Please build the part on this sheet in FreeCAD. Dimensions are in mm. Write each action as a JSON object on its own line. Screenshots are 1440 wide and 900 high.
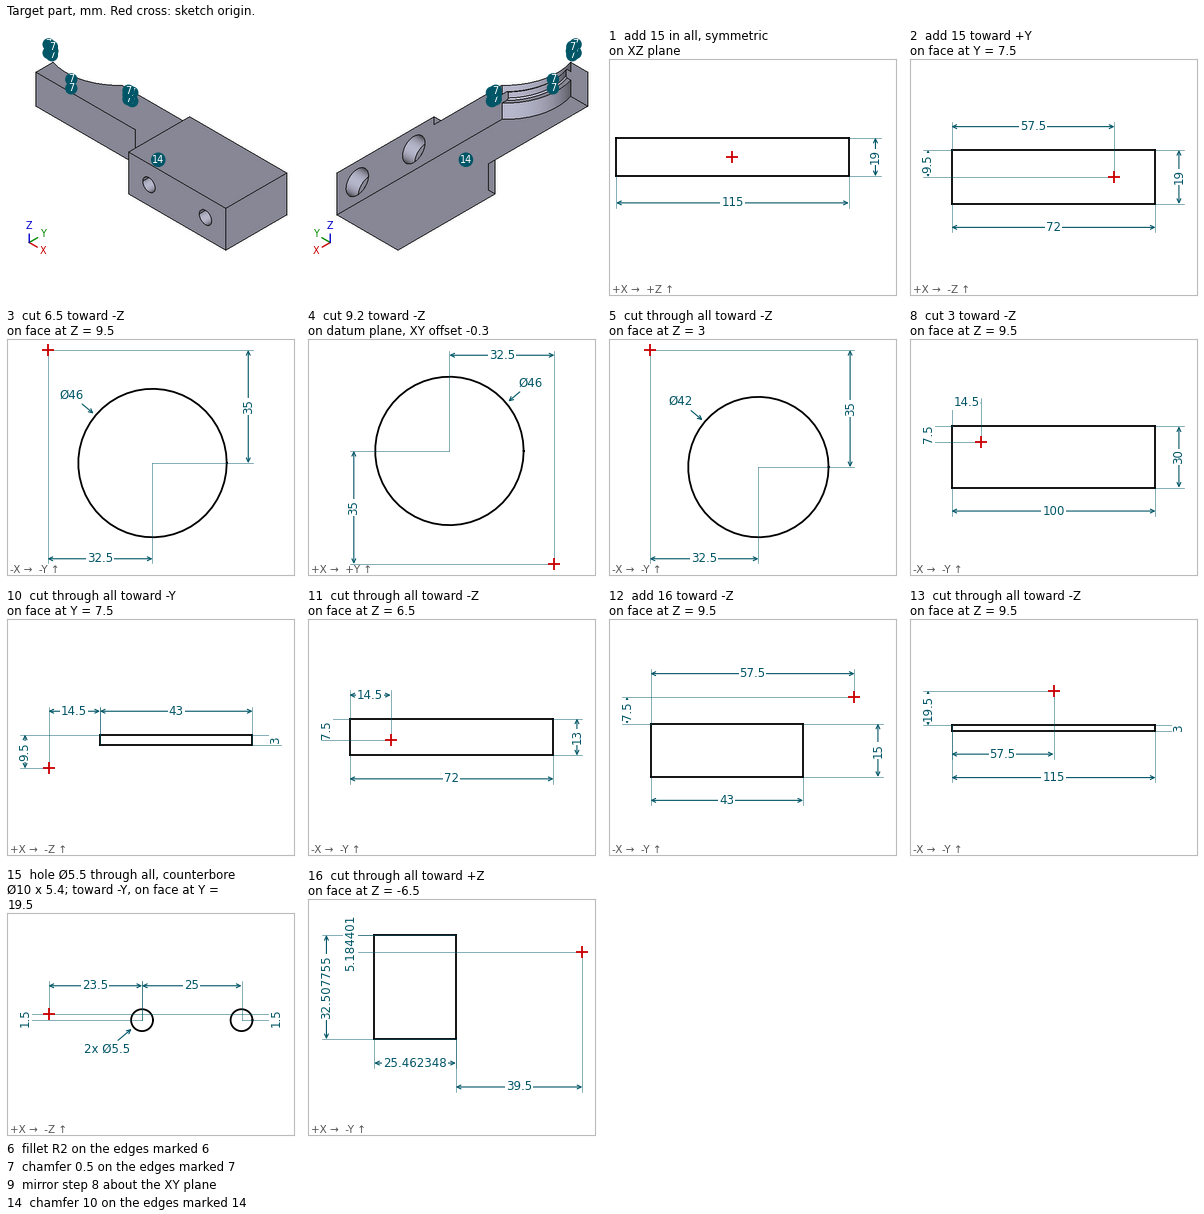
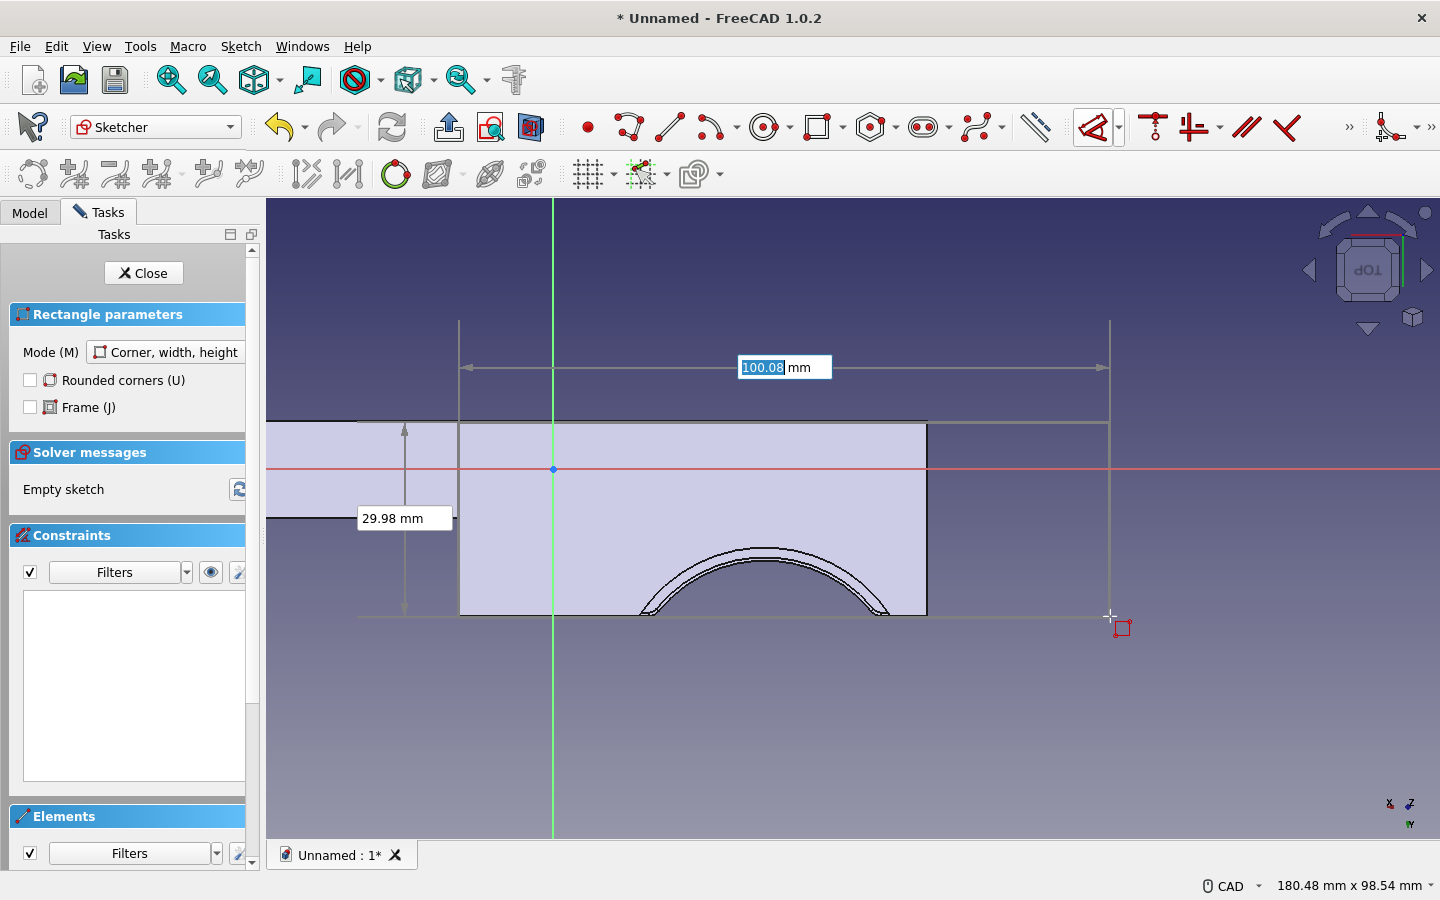
{"action": "type", "text": "100"}
{"action": "key", "text": "Tab"}
{"action": "type", "text": "30"}
{"action": "key", "text": "Return"}
{"action": "key", "text": "Escape"}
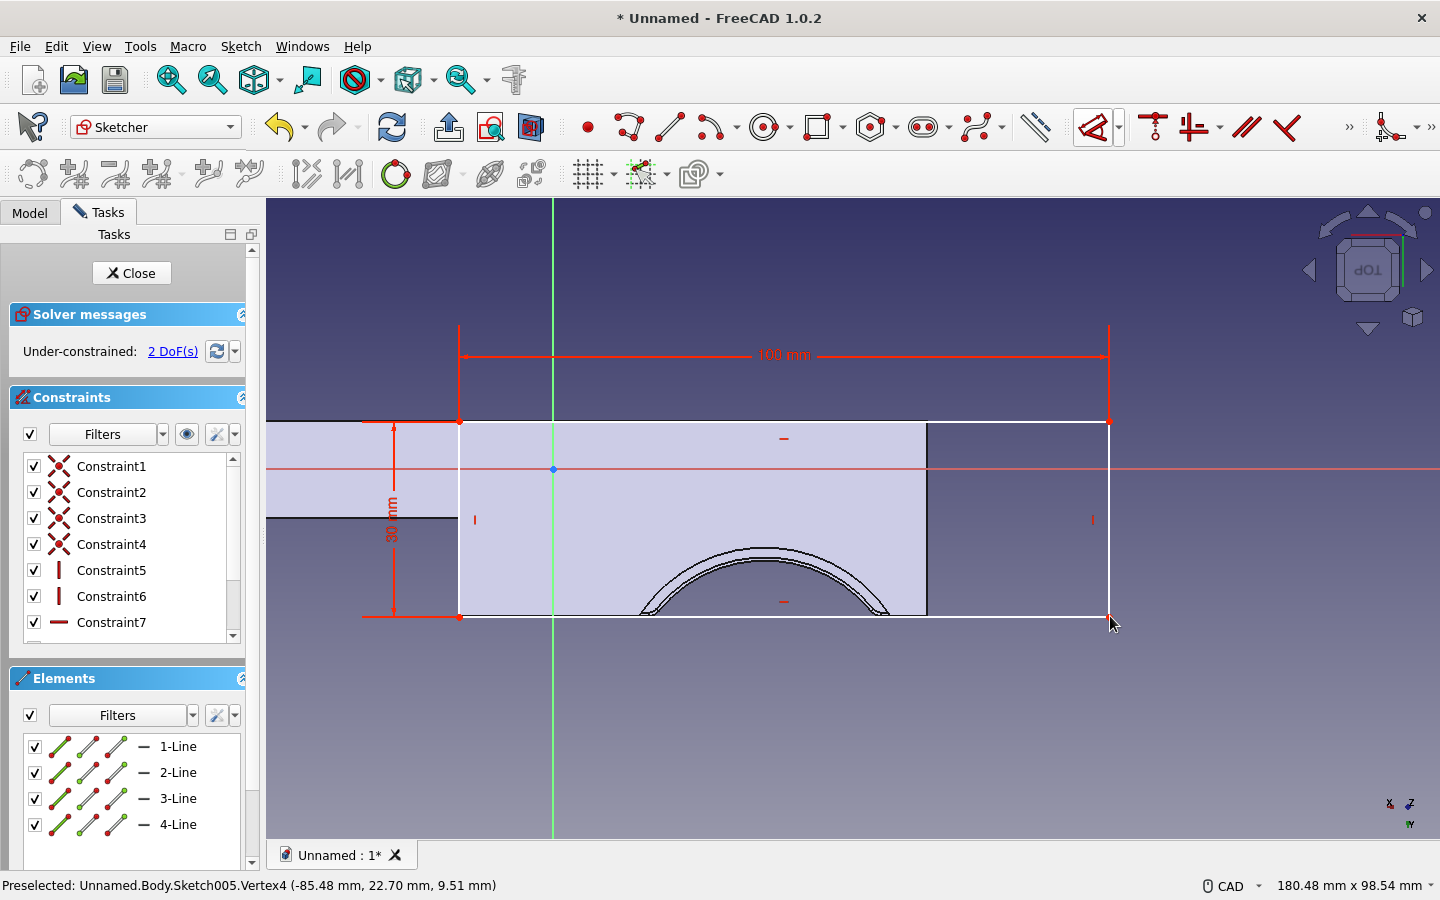
{"action": "left_click", "coordinate": [459, 422]}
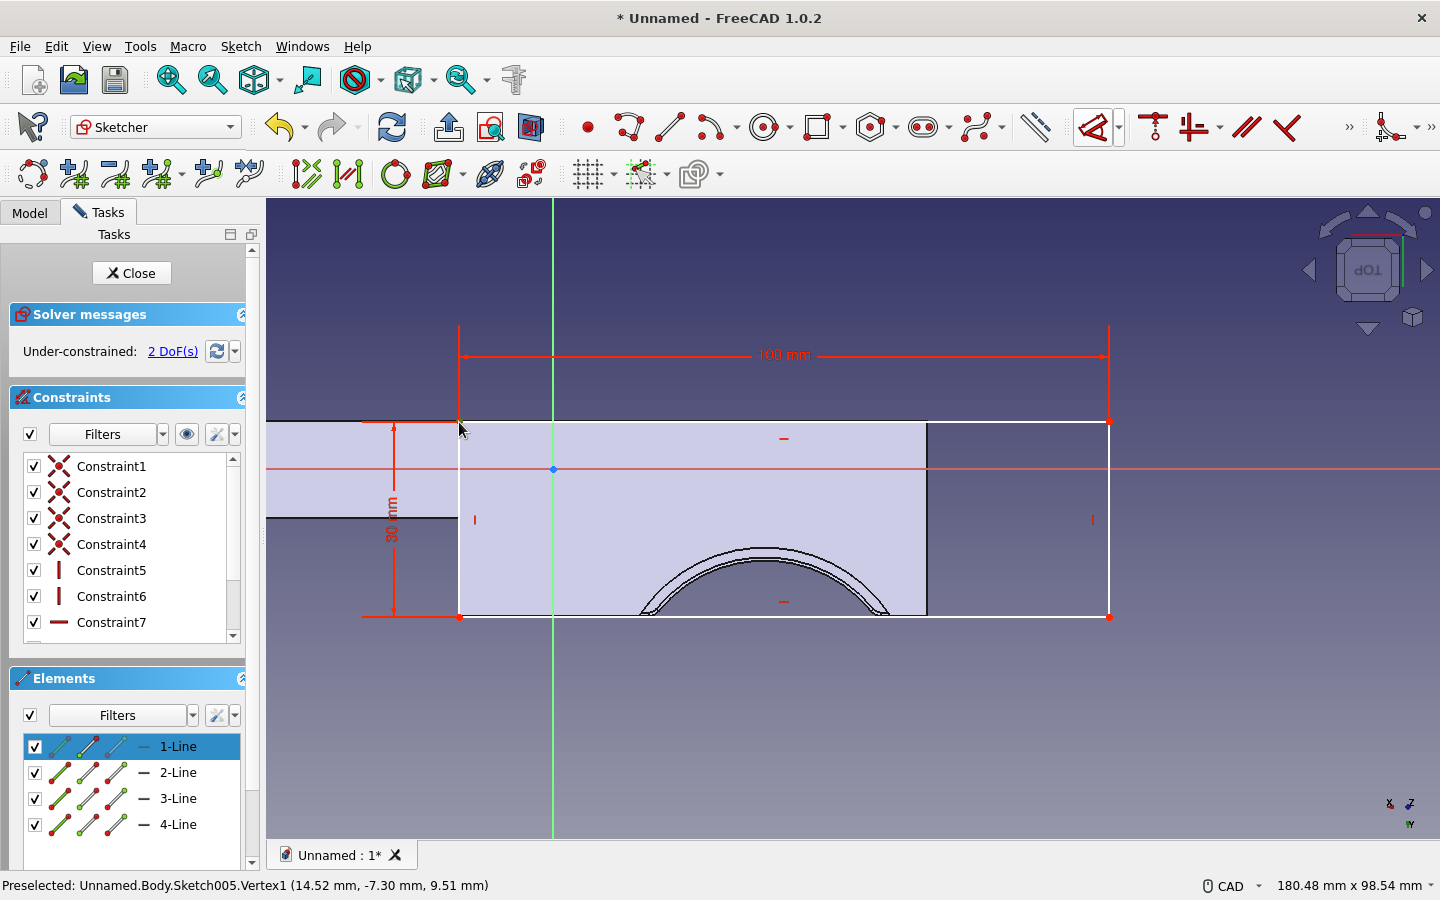
{"action": "left_click", "coordinate": [1118, 128]}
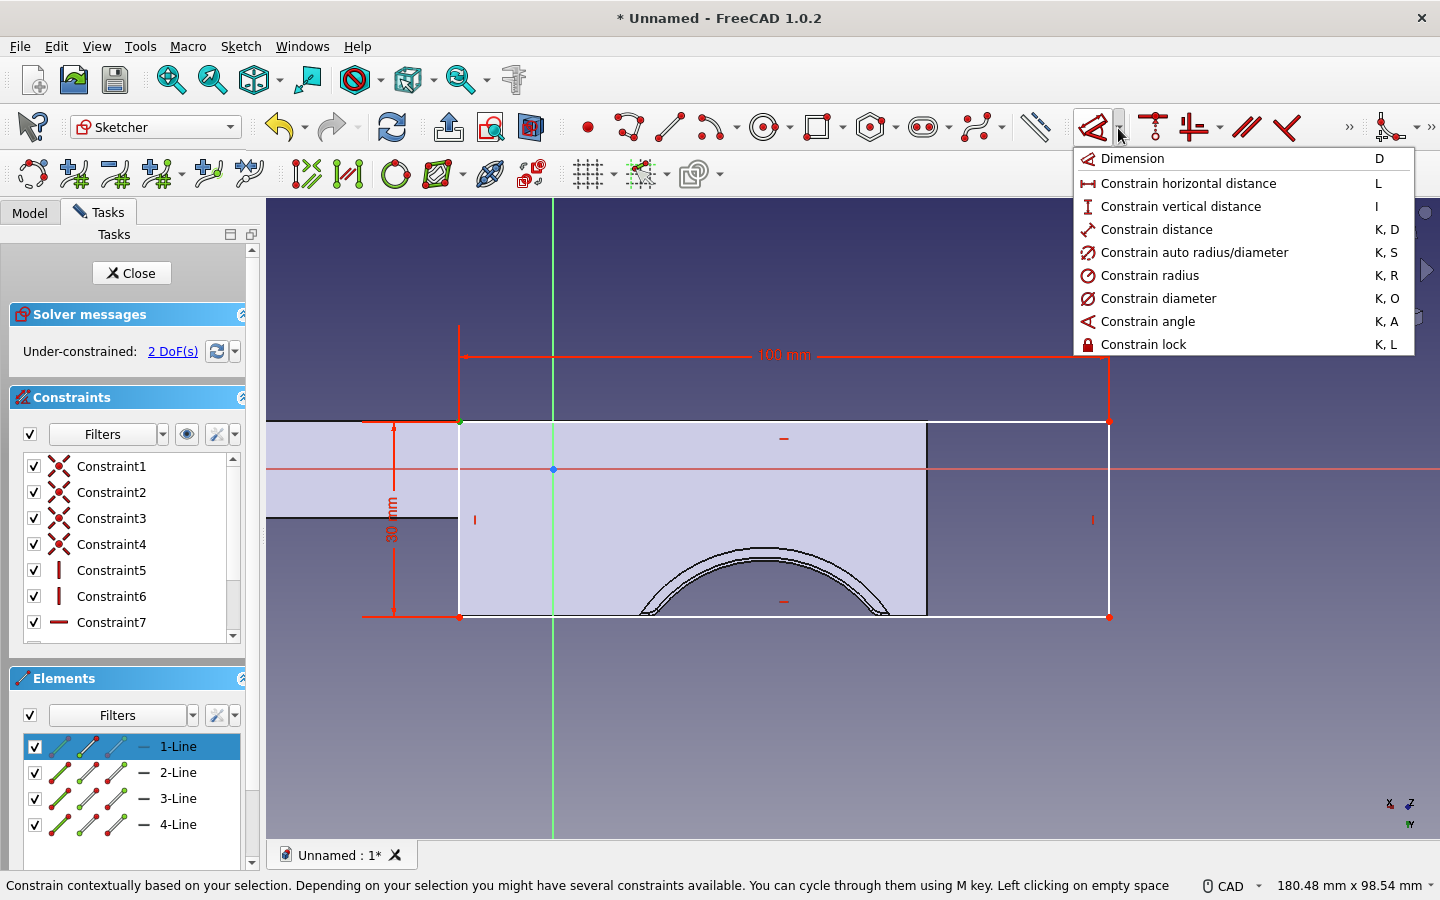
{"action": "left_click", "coordinate": [1244, 206]}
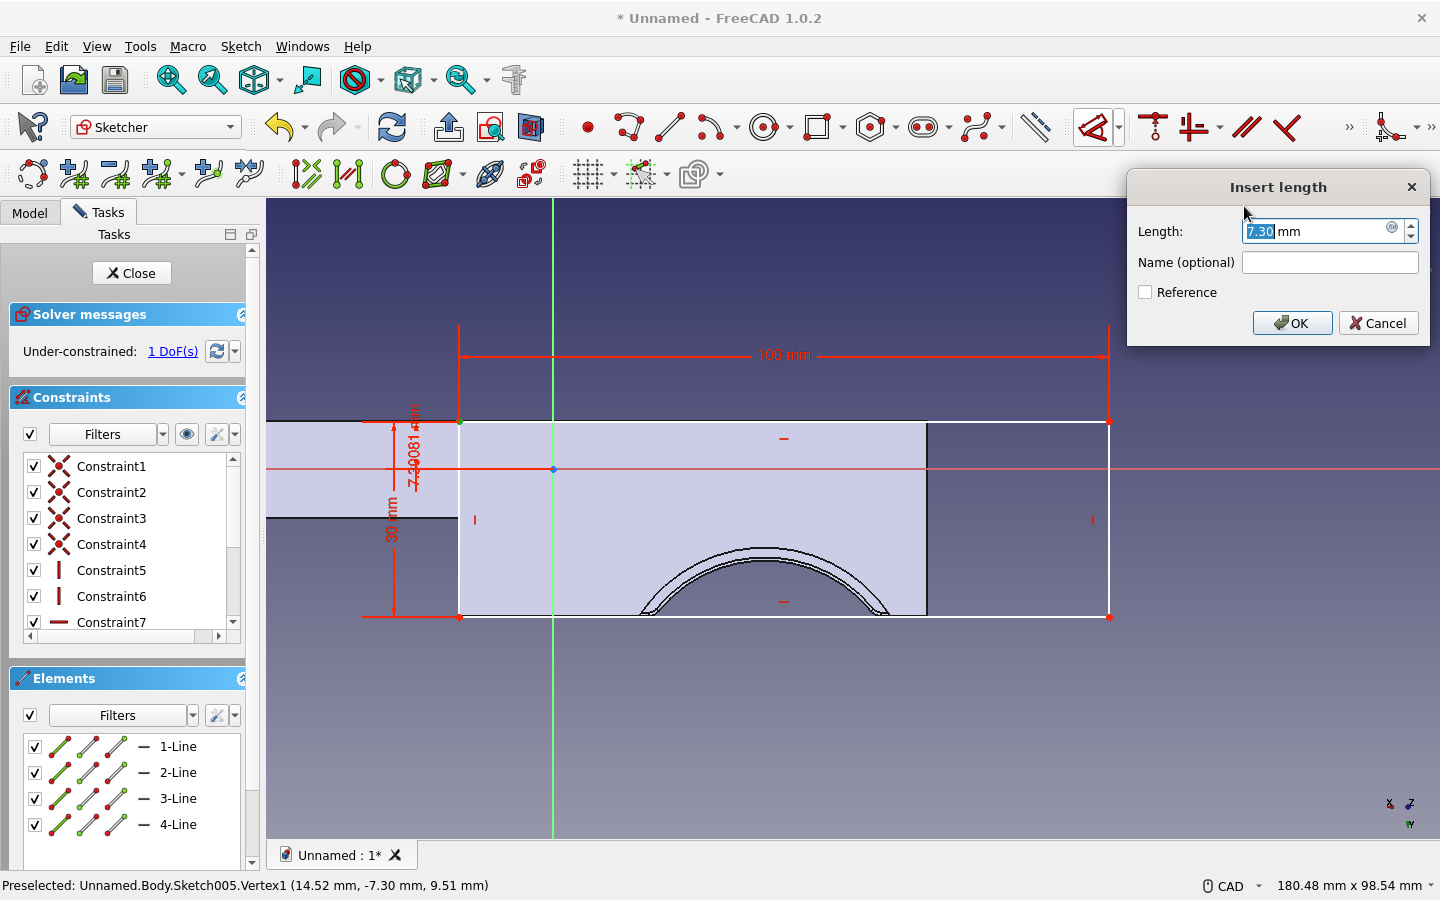
{"action": "type", "text": "7.5"}
{"action": "key", "text": "Return"}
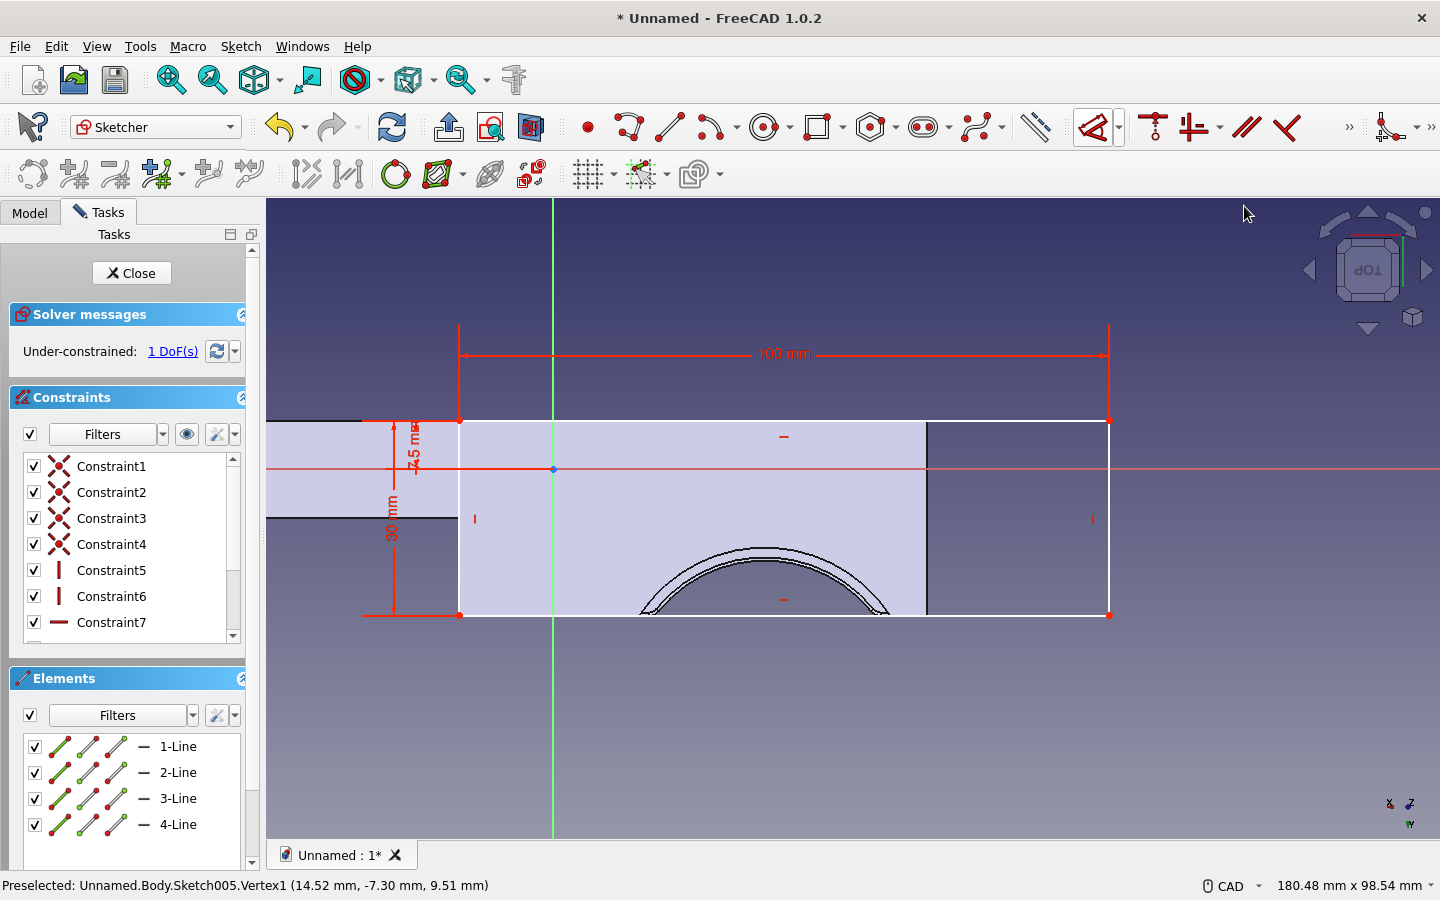
{"action": "left_click", "coordinate": [459, 421]}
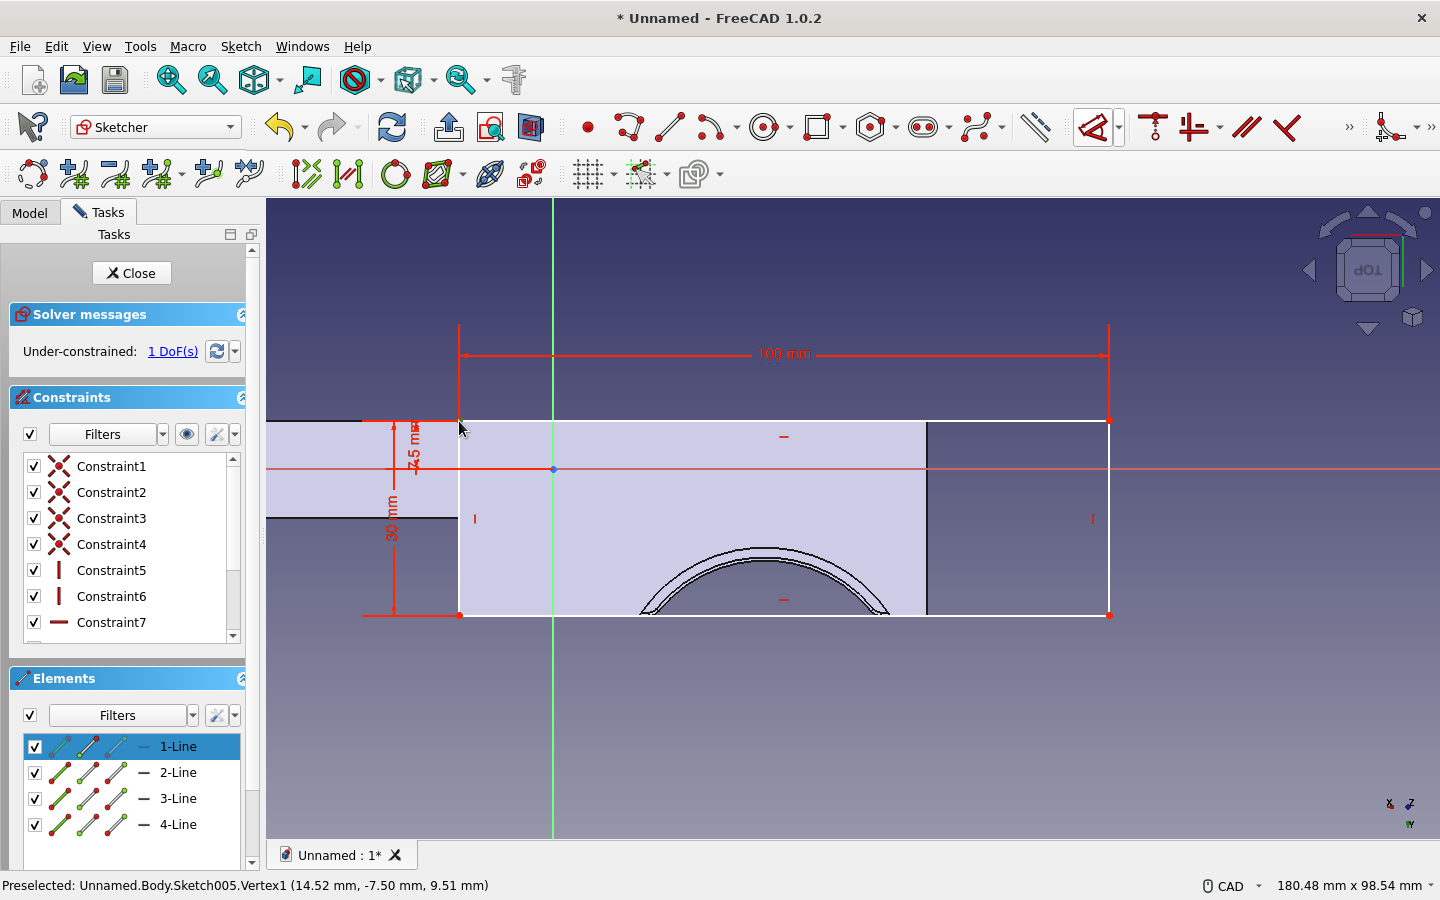
{"action": "key", "text": "l"}